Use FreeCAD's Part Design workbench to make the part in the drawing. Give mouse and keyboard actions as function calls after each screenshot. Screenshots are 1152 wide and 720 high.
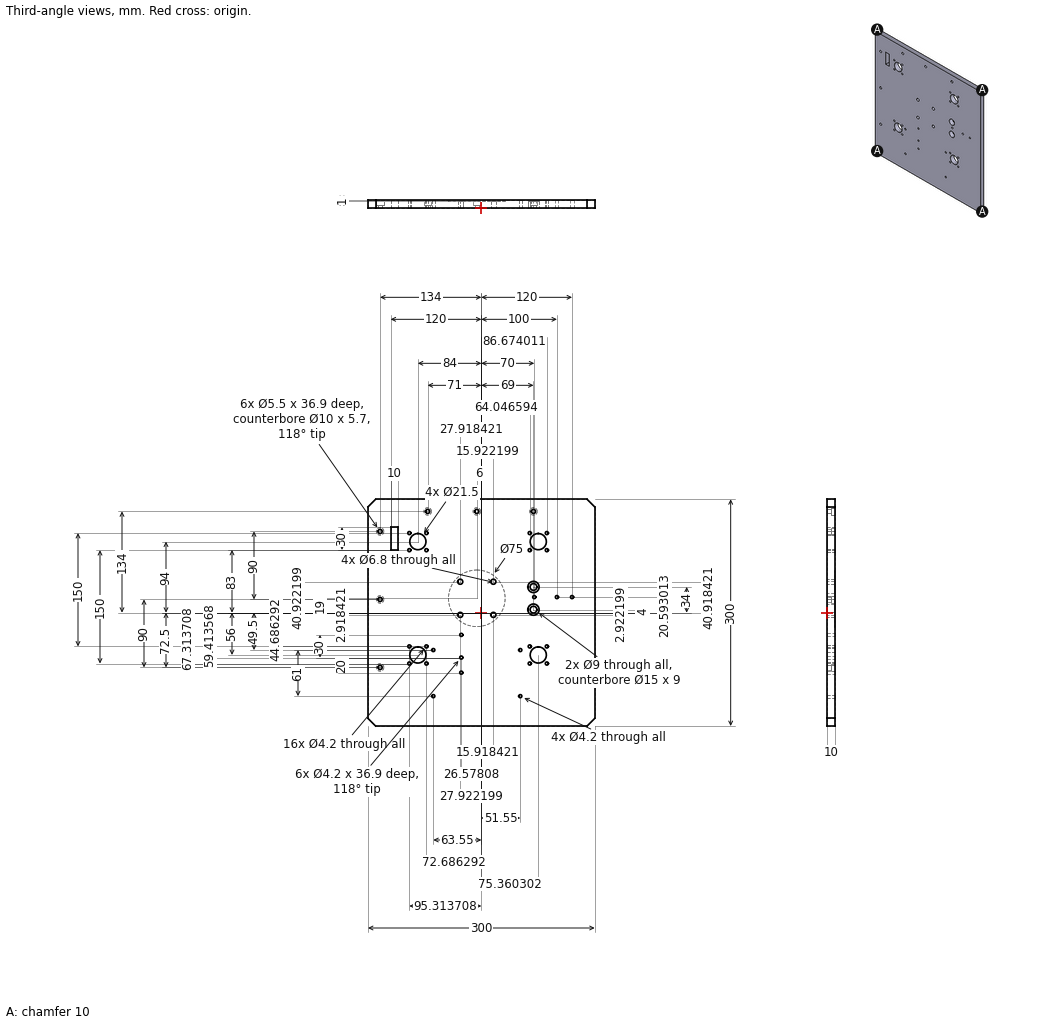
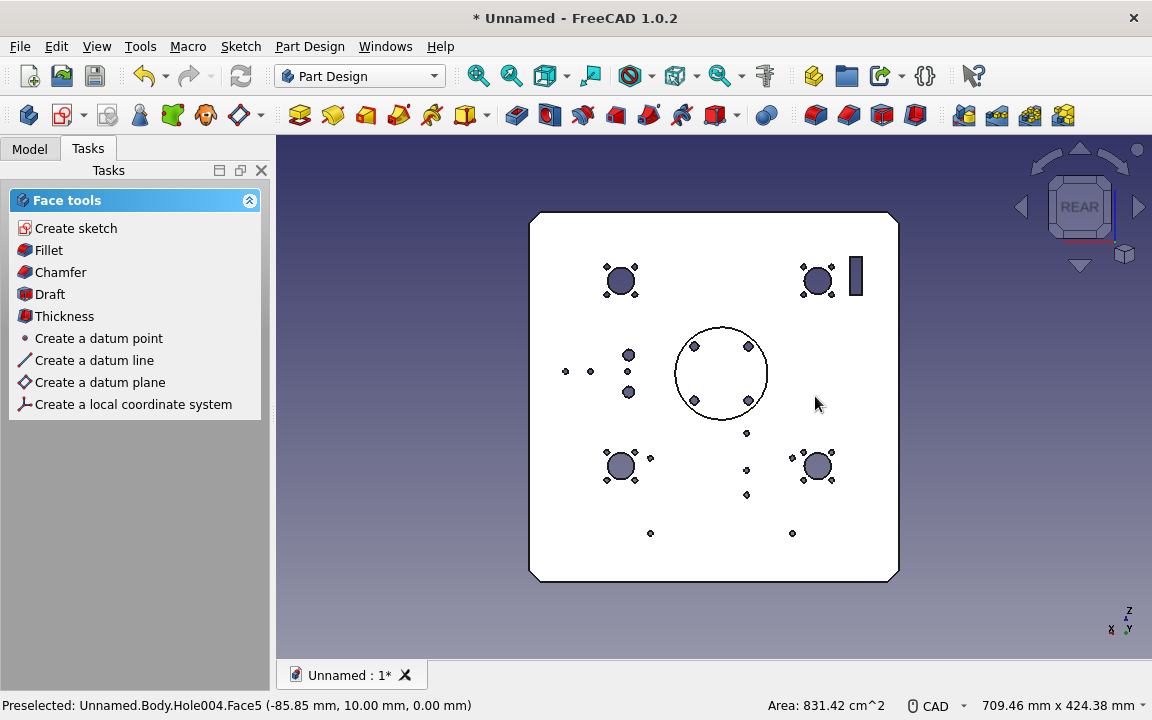
click(62, 116)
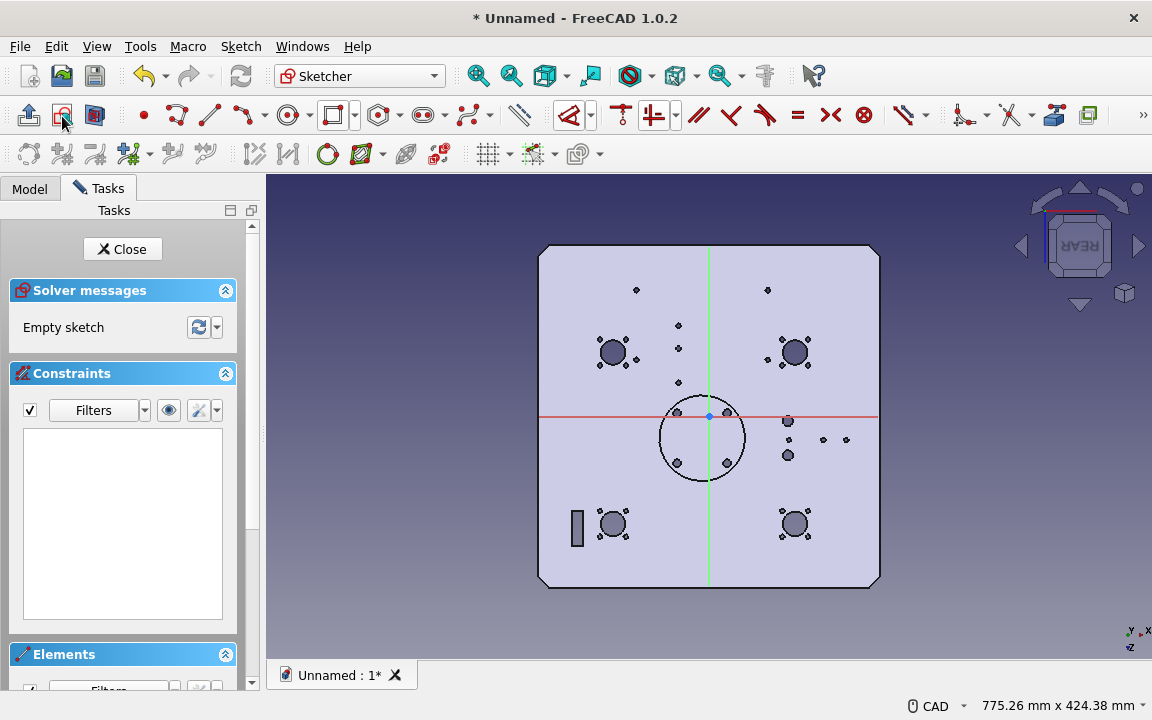
click(288, 116)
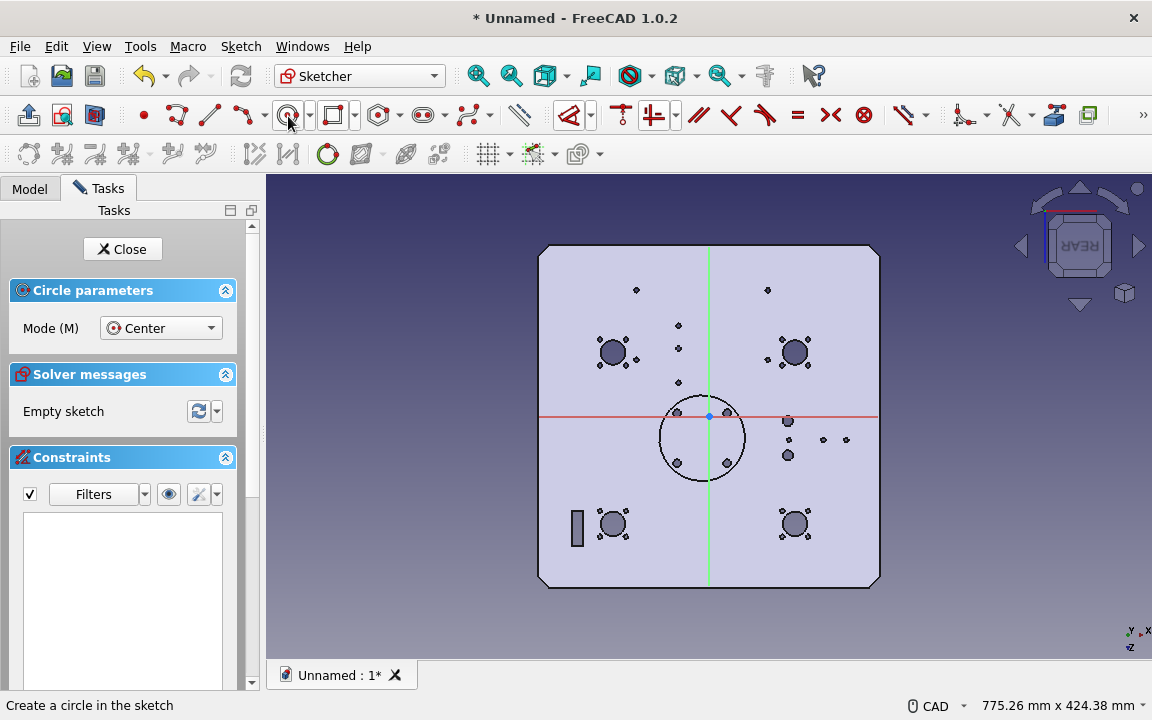
scroll(556, 539, up, 10)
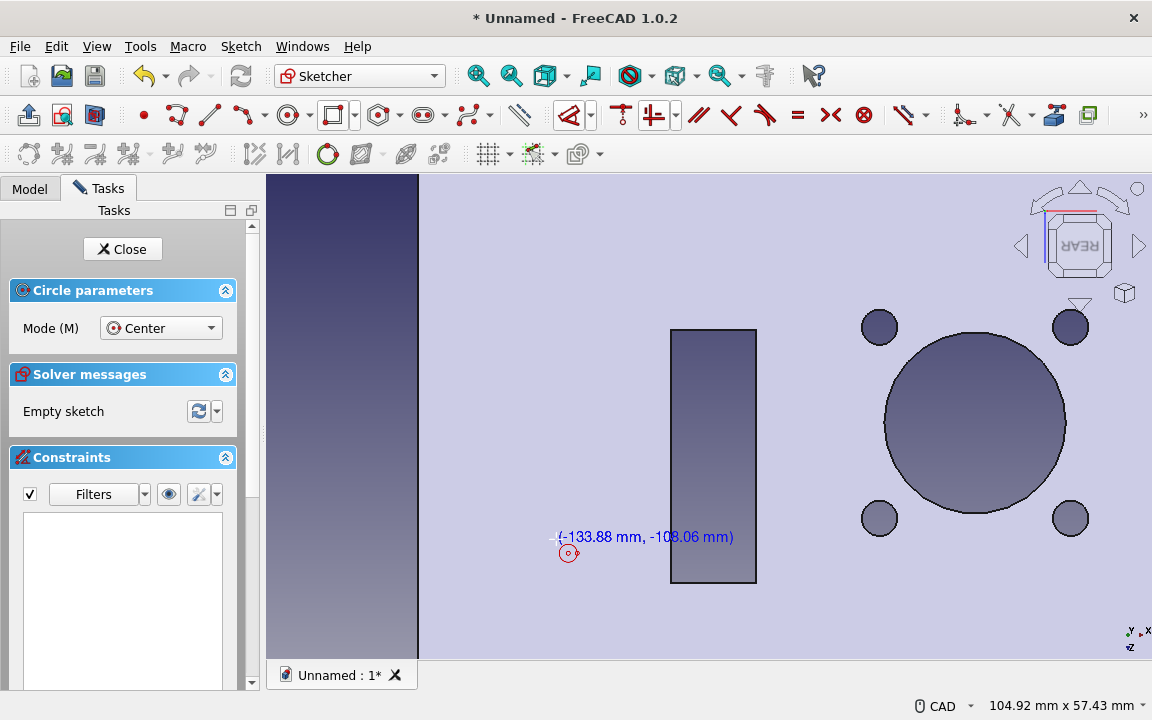
scroll(488, 521, down, 9)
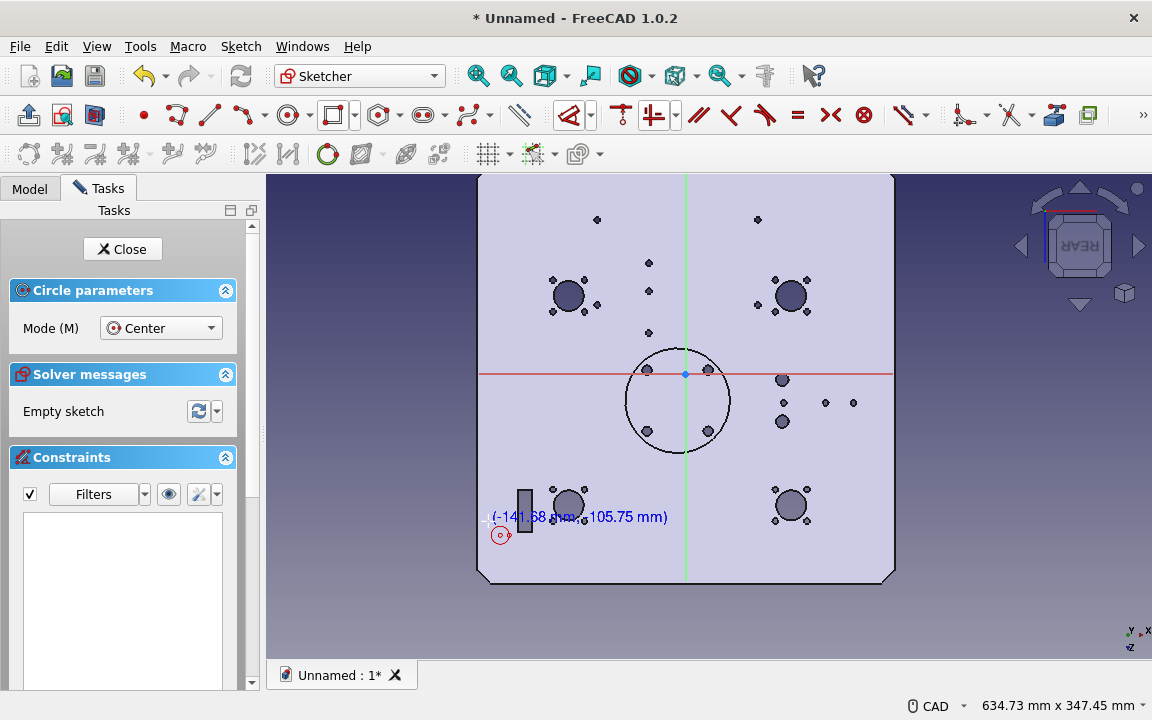
click(499, 524)
move(502, 521)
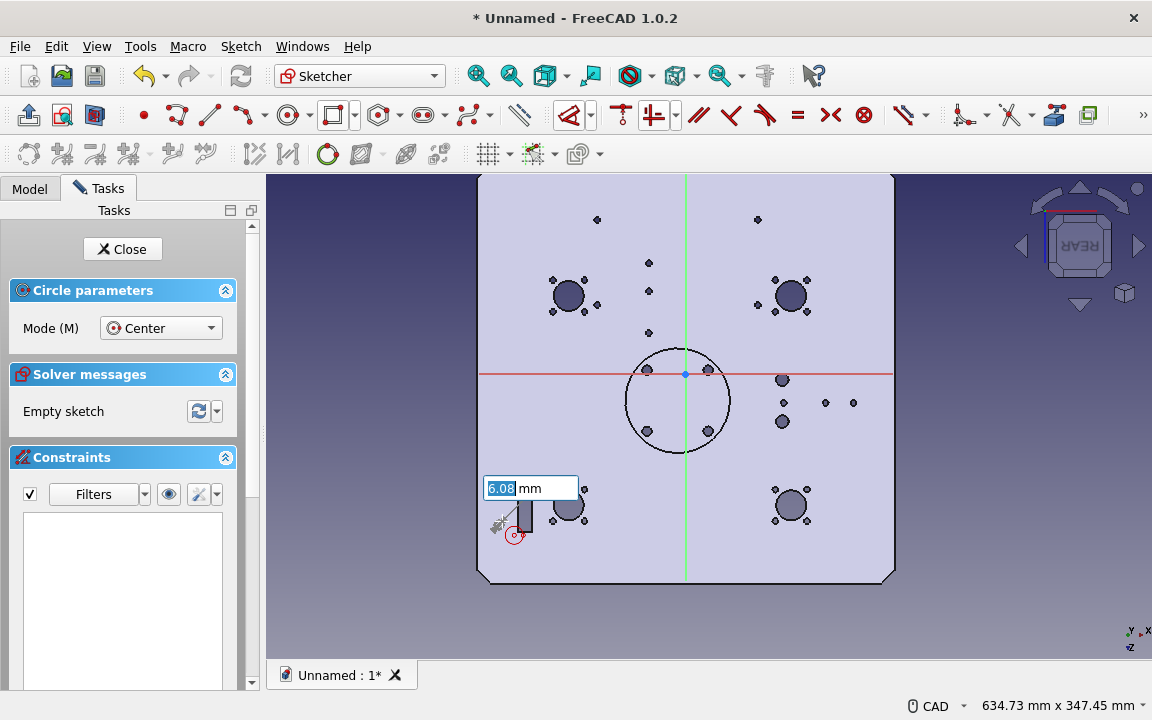
text(5.5)
key(Return)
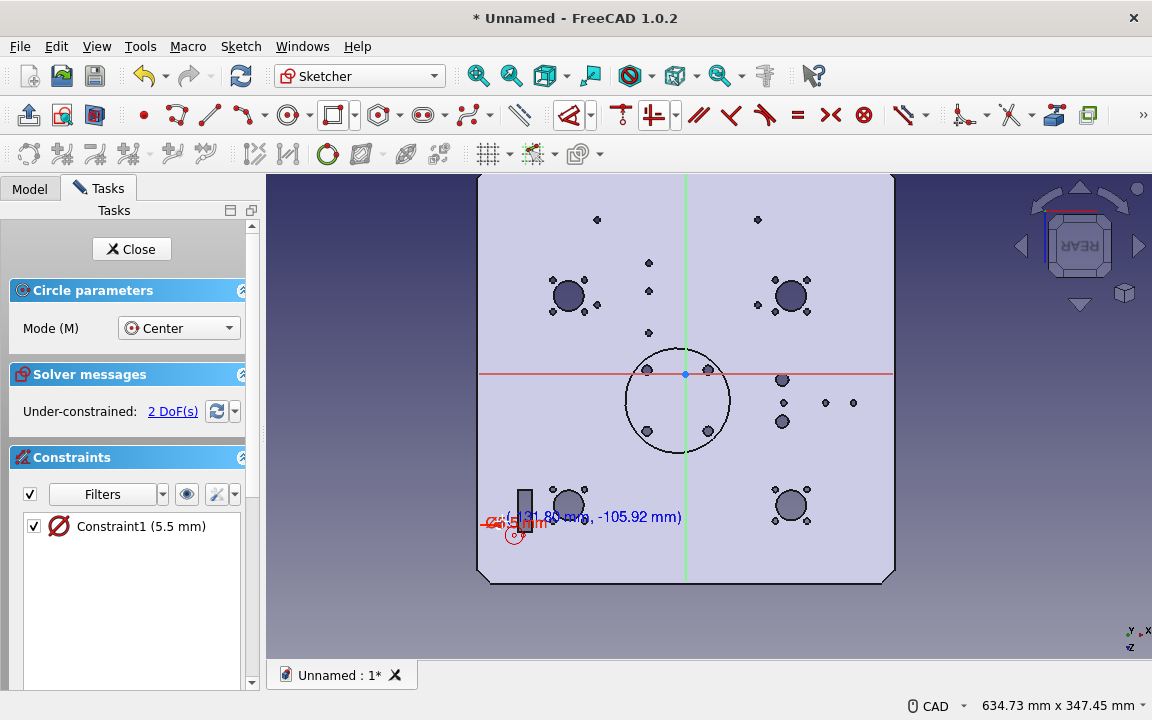
scroll(587, 561, up, 9)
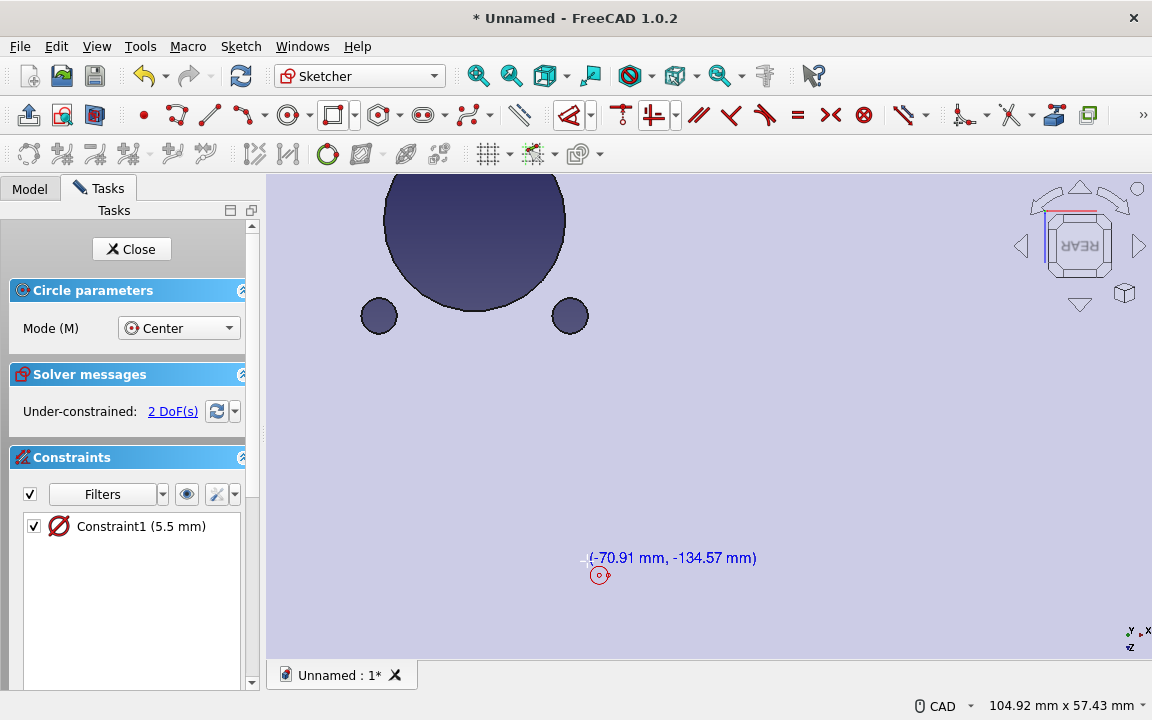
scroll(587, 561, down, 9)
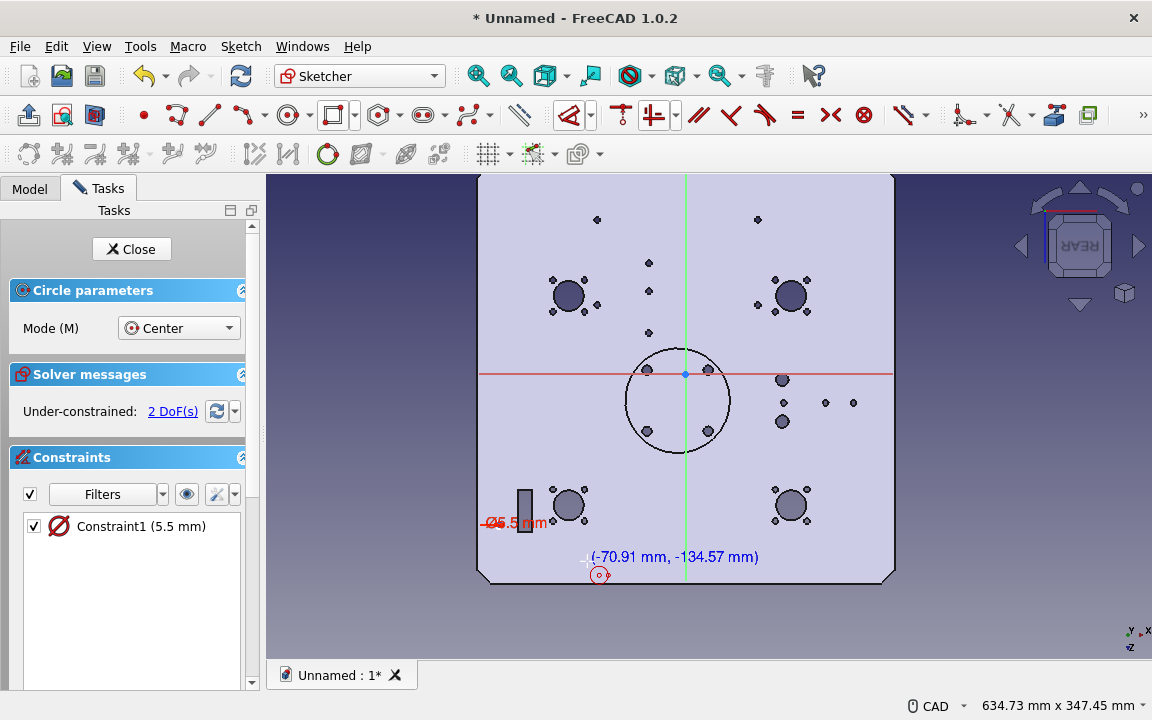
click(587, 561)
move(590, 558)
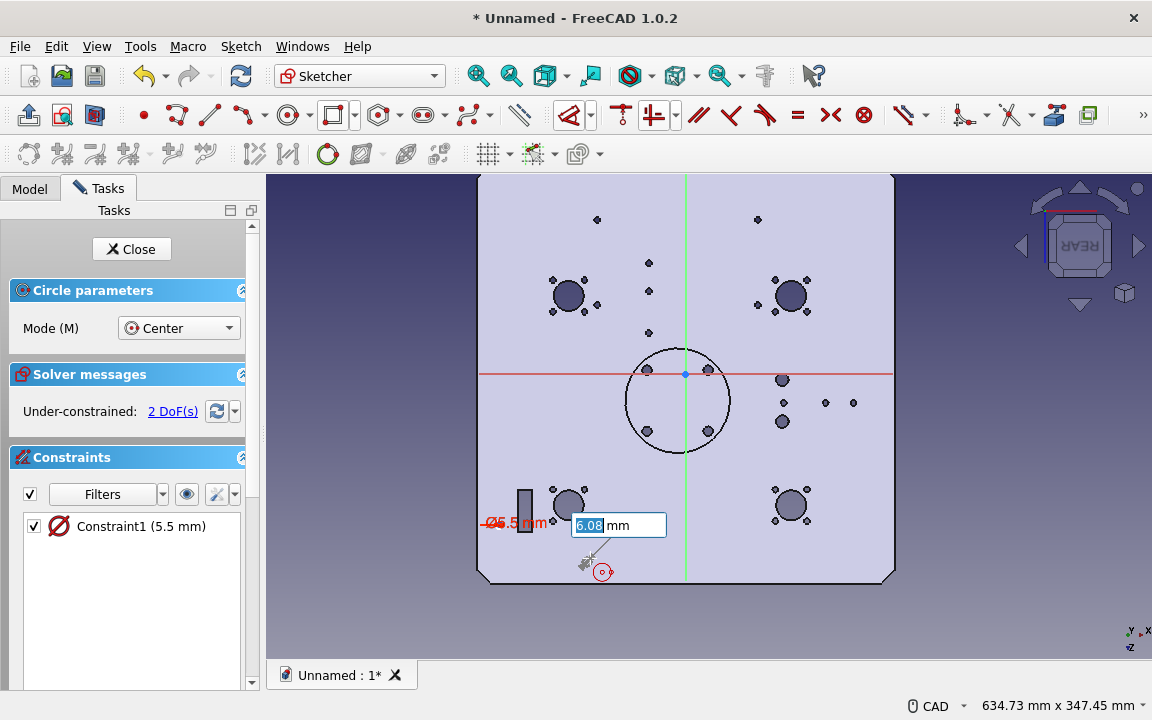
text(5.5)
key(Return)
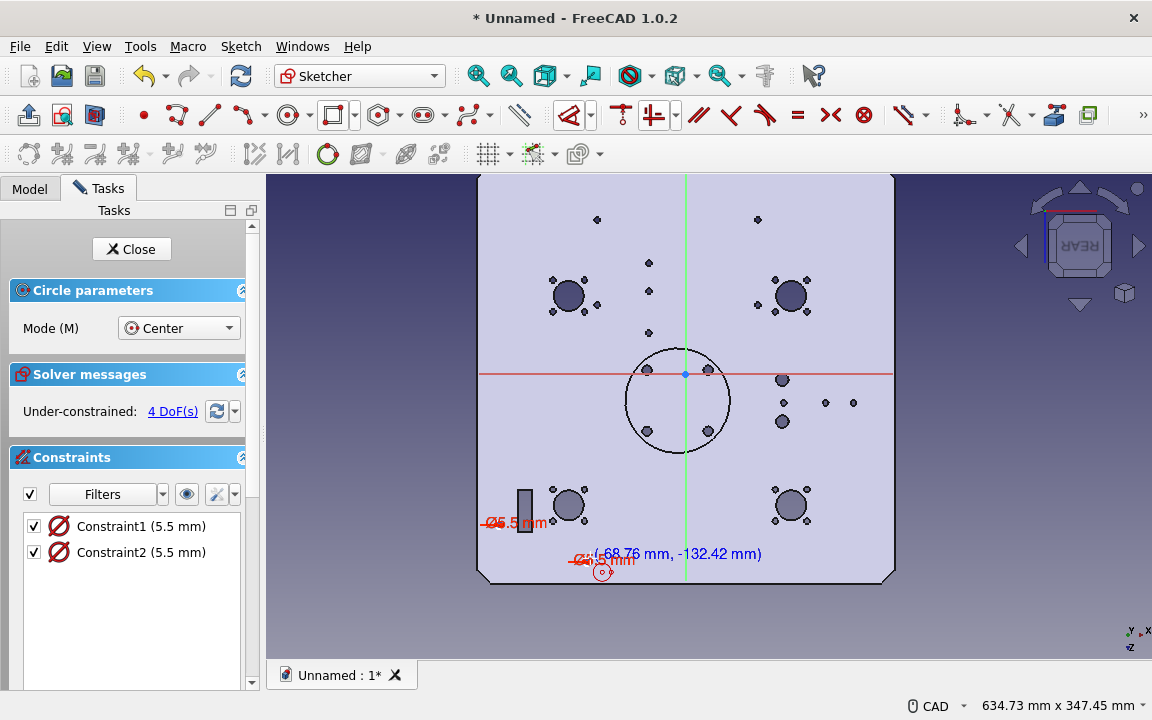
scroll(678, 561, up, 9)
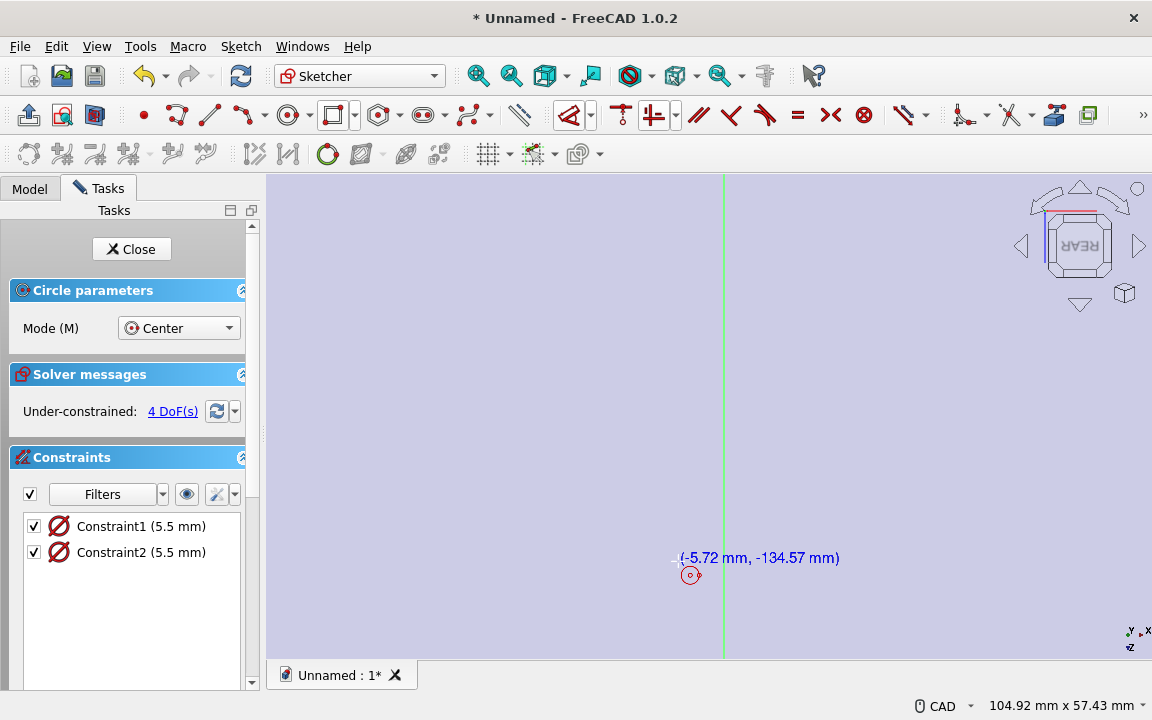
scroll(678, 561, down, 9)